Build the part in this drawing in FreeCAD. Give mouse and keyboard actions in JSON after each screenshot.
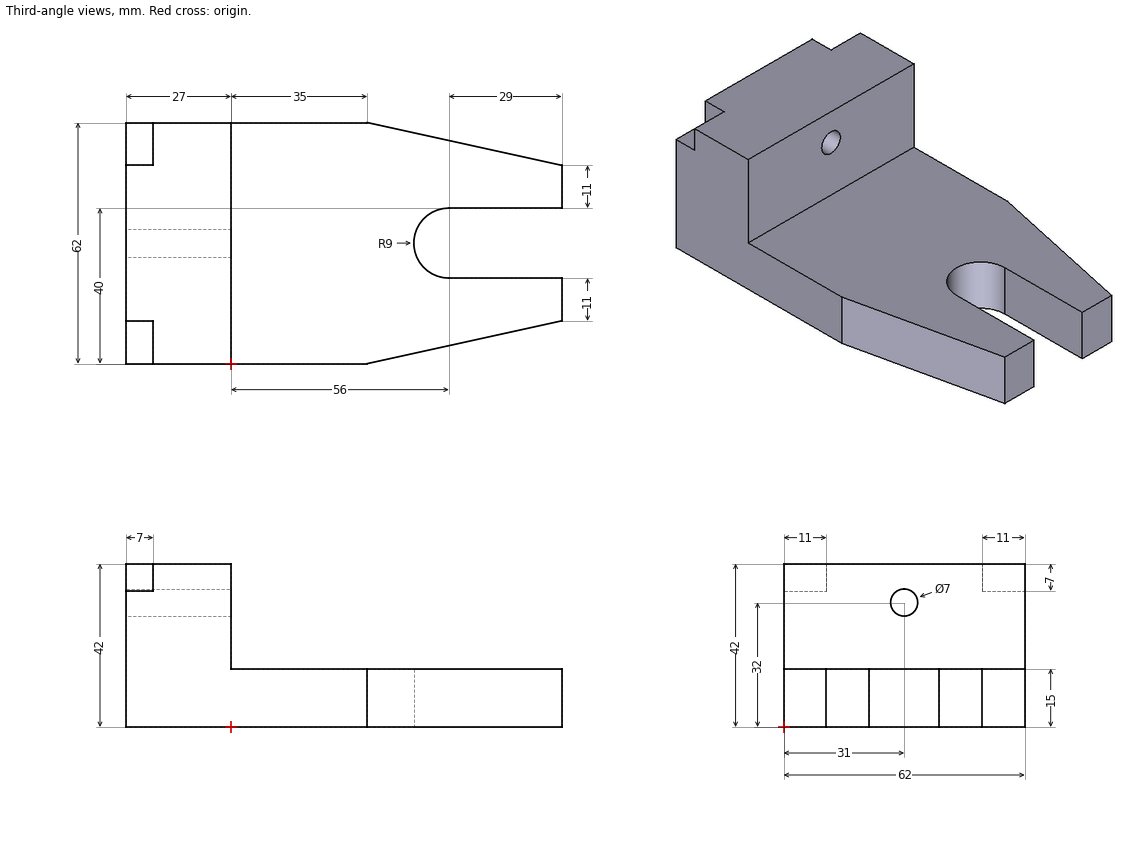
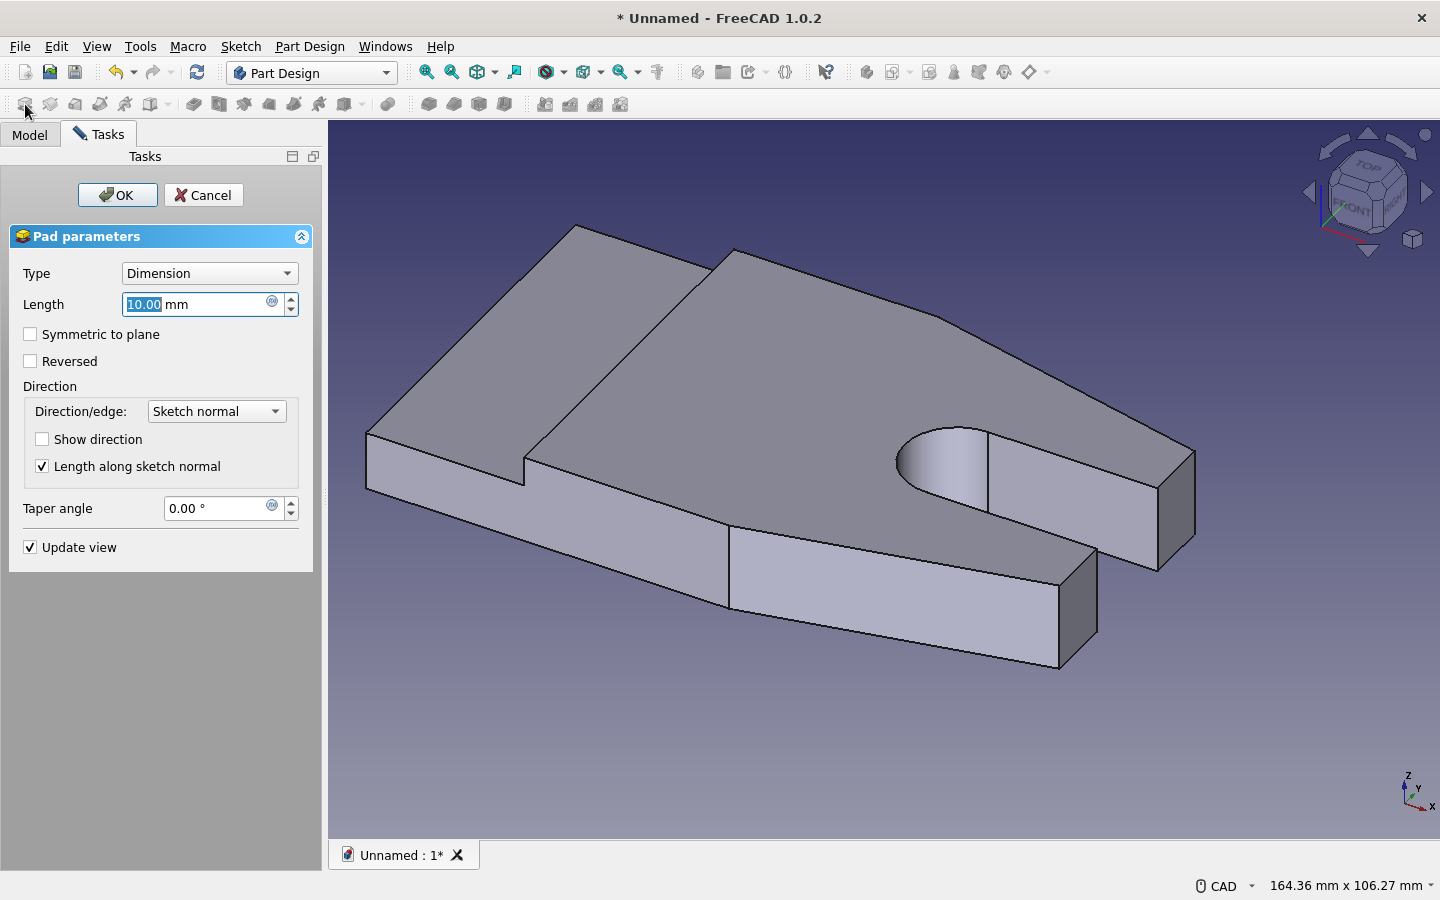
{"action": "type", "text": "42"}
{"action": "key", "text": "Tab"}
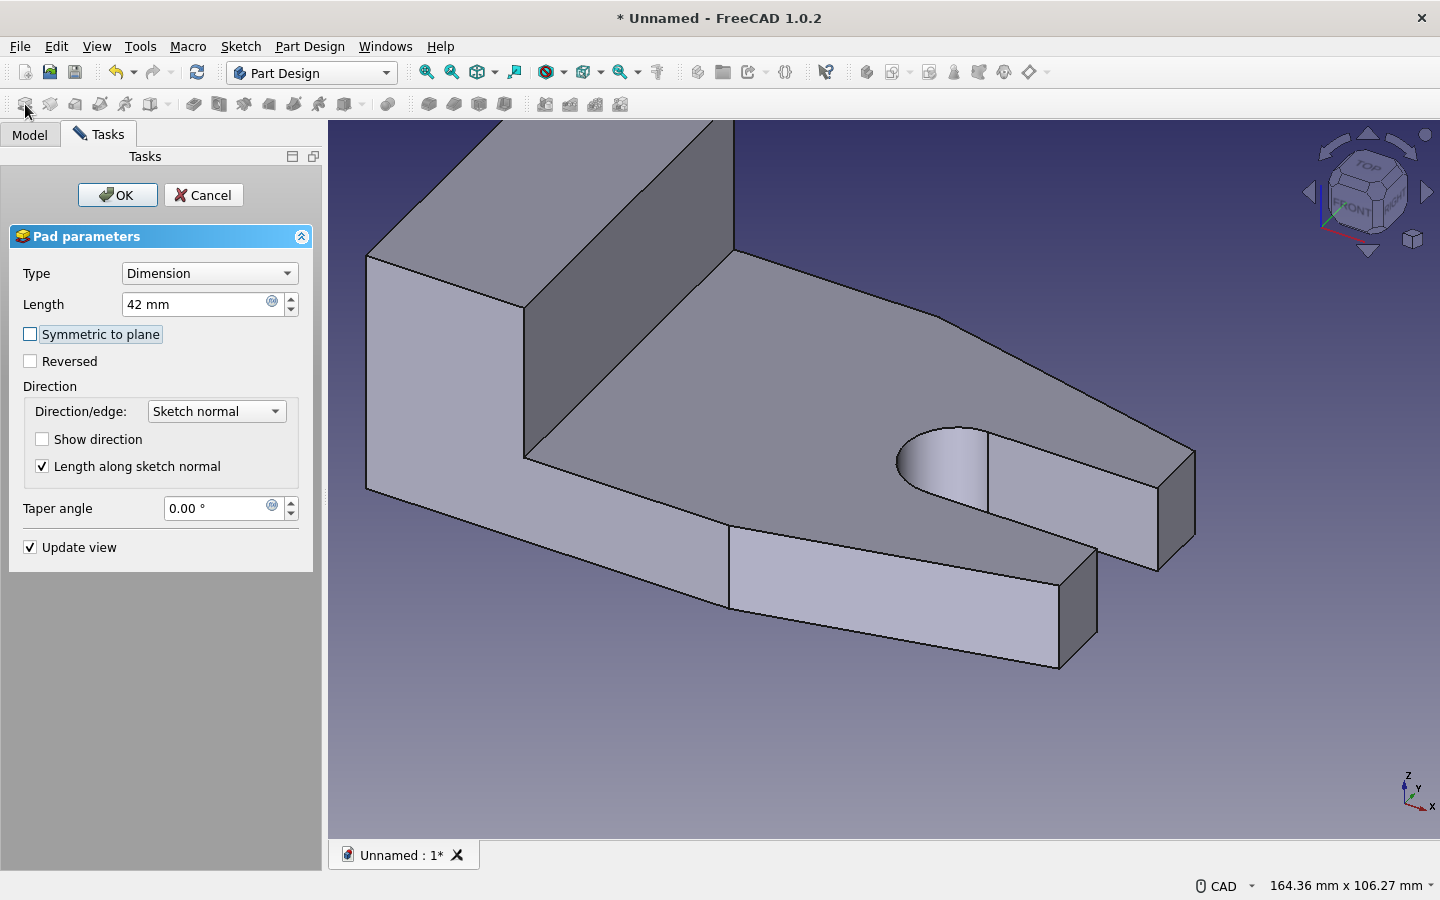
{"action": "left_click", "coordinate": [118, 195]}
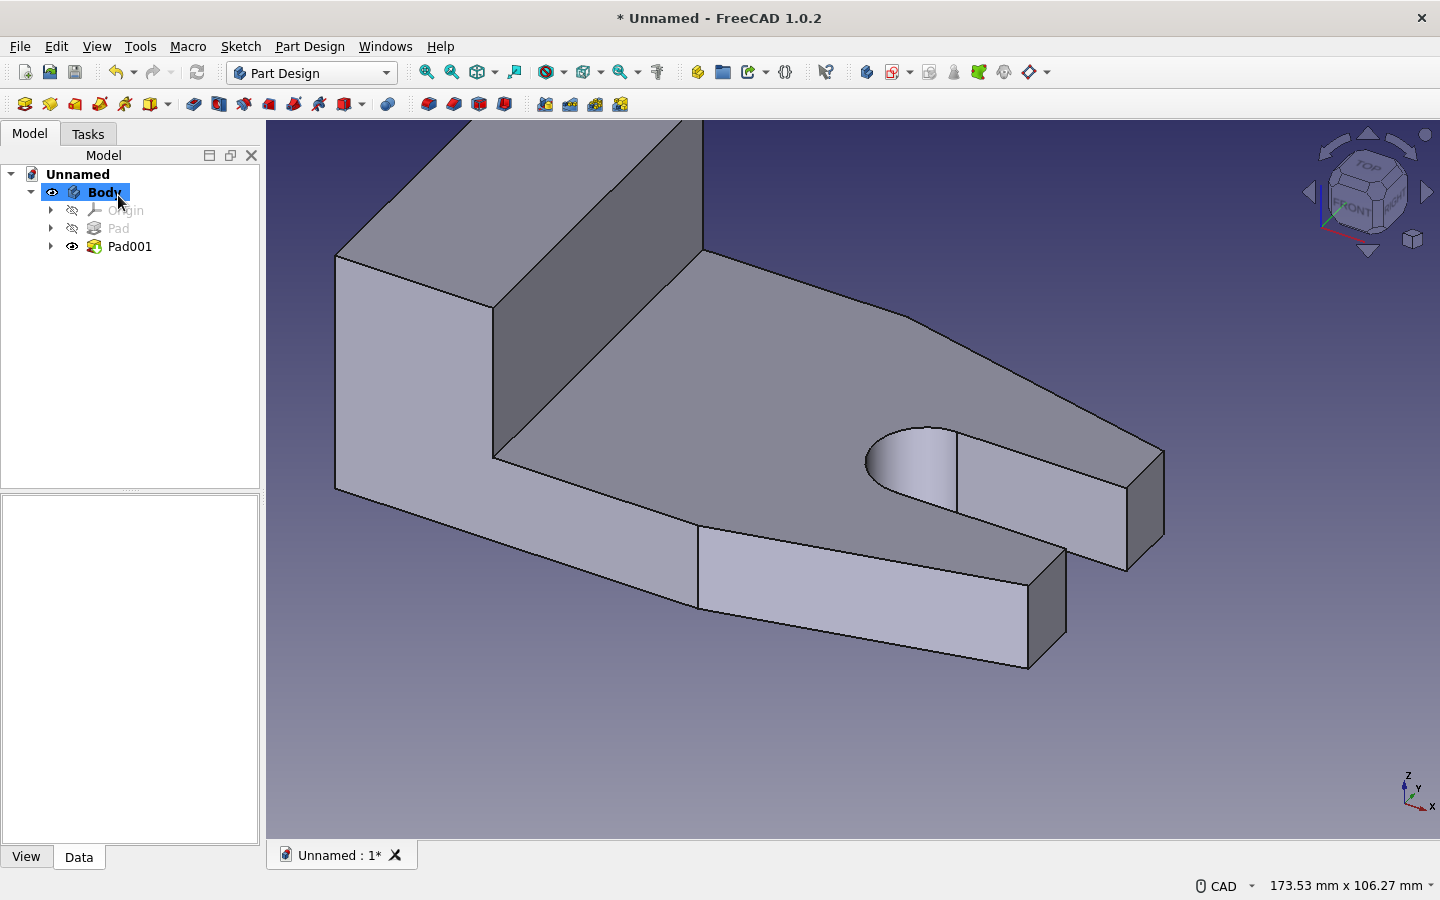
{"action": "left_click", "coordinate": [427, 72]}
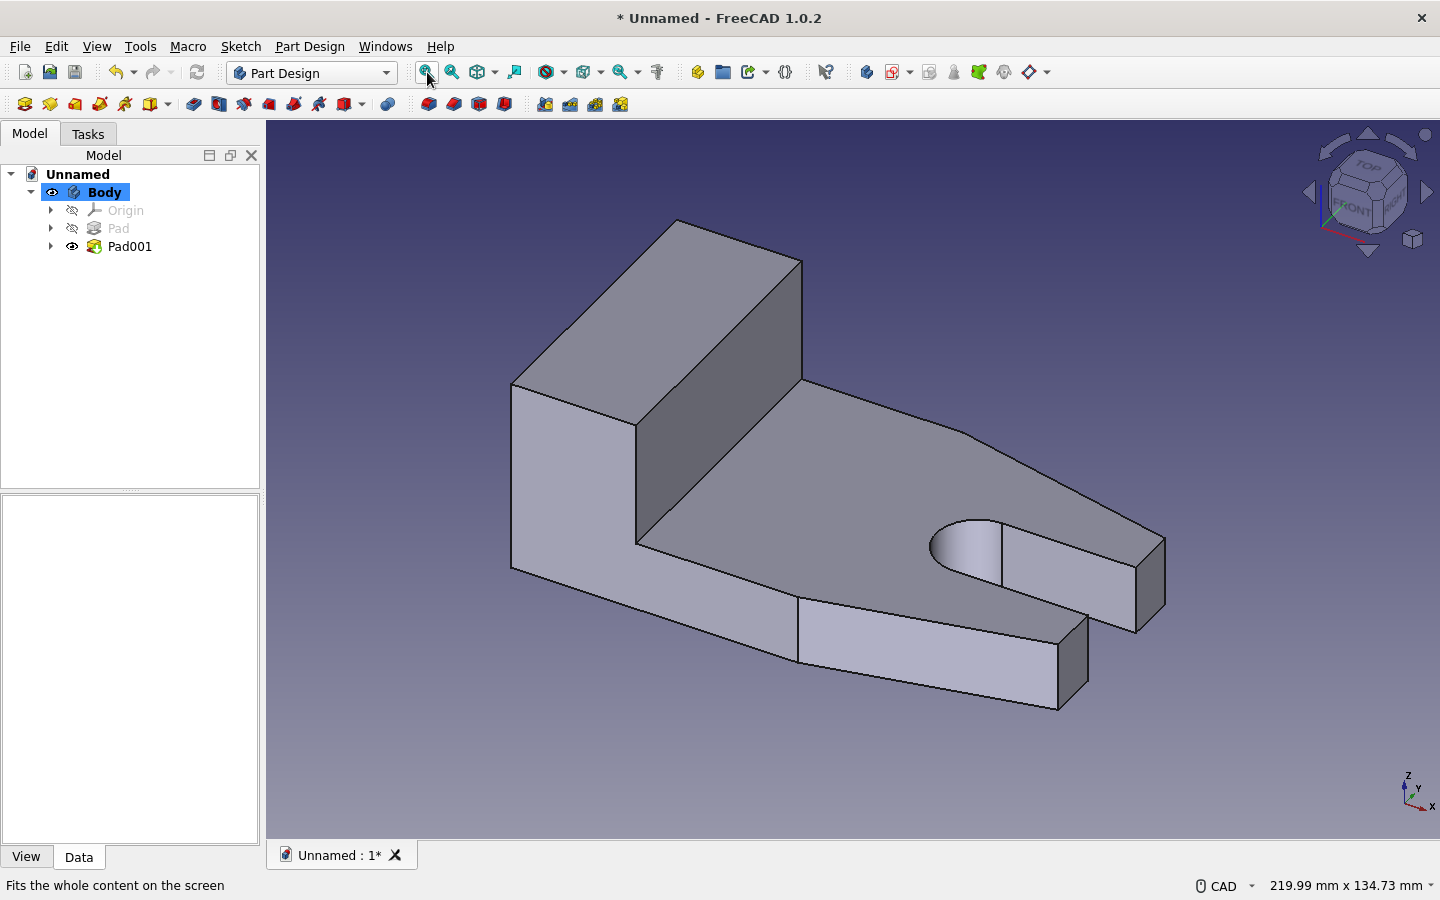
{"action": "key", "text": "6"}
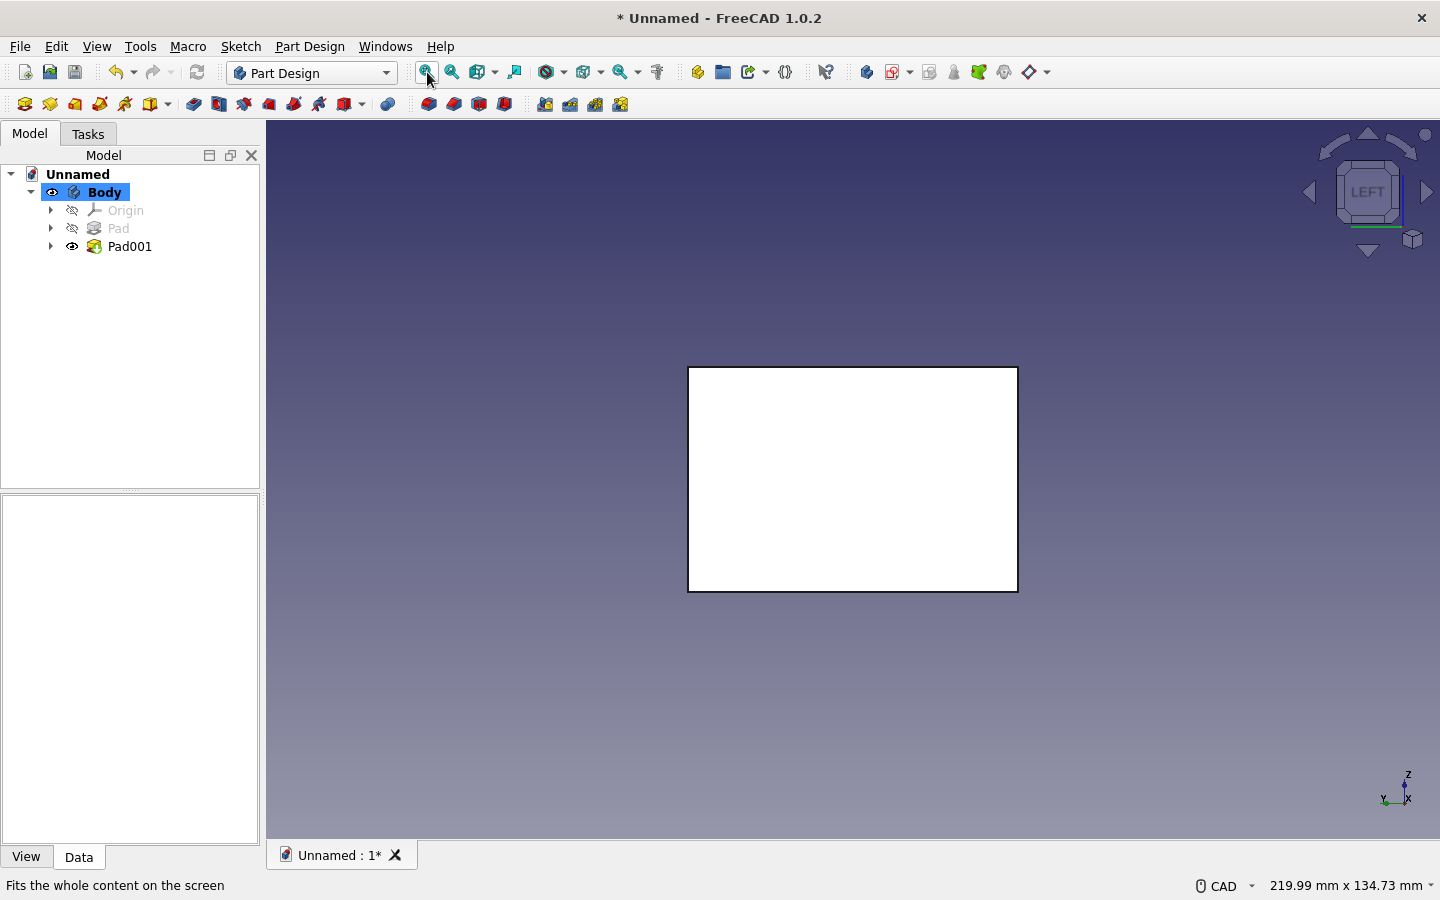
{"action": "left_click", "coordinate": [427, 72]}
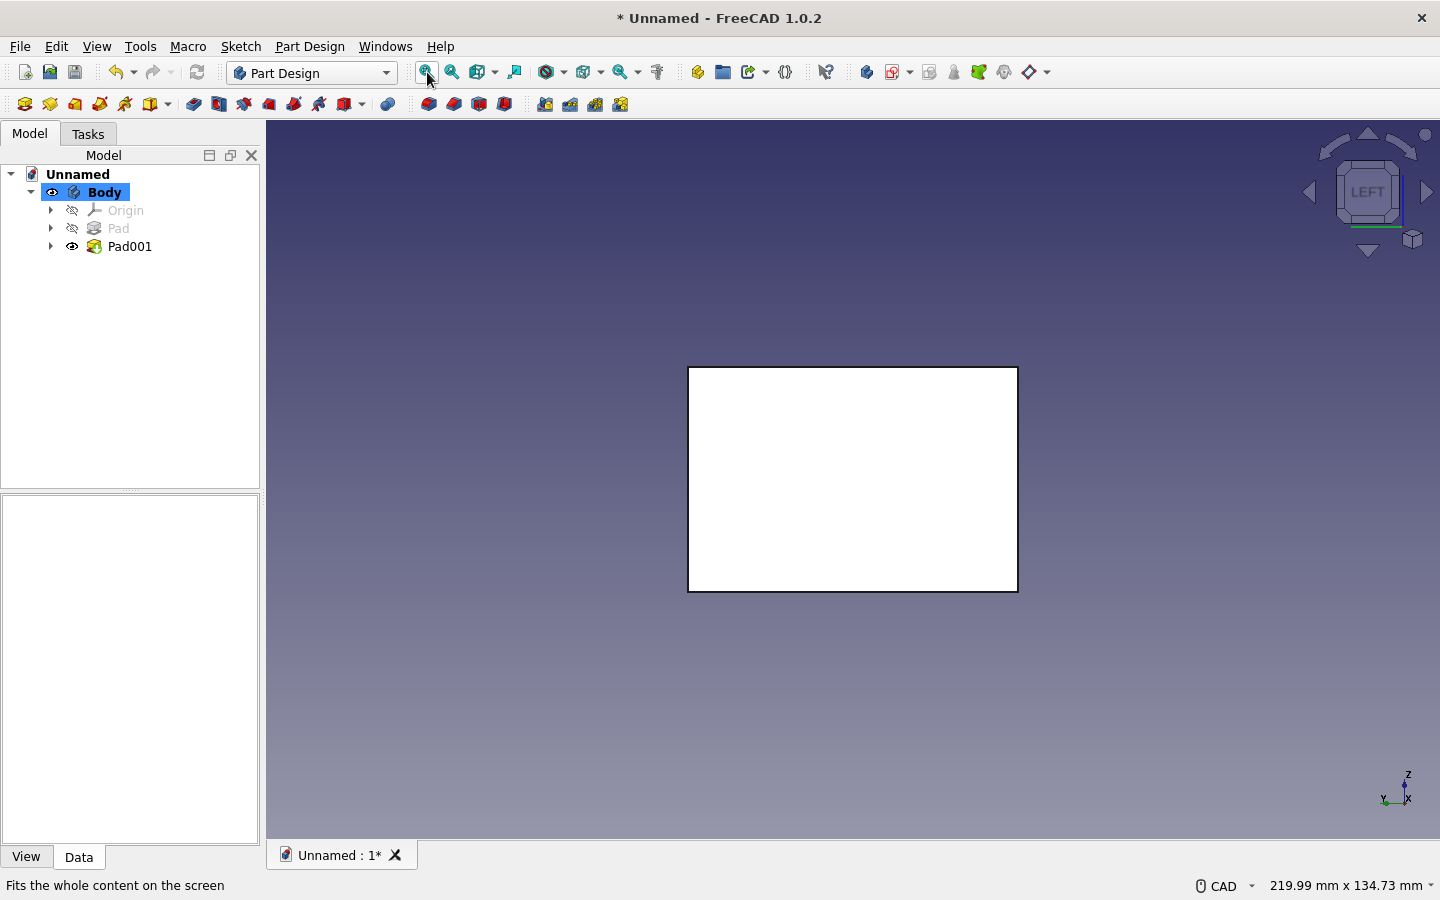
{"action": "left_click", "coordinate": [806, 478]}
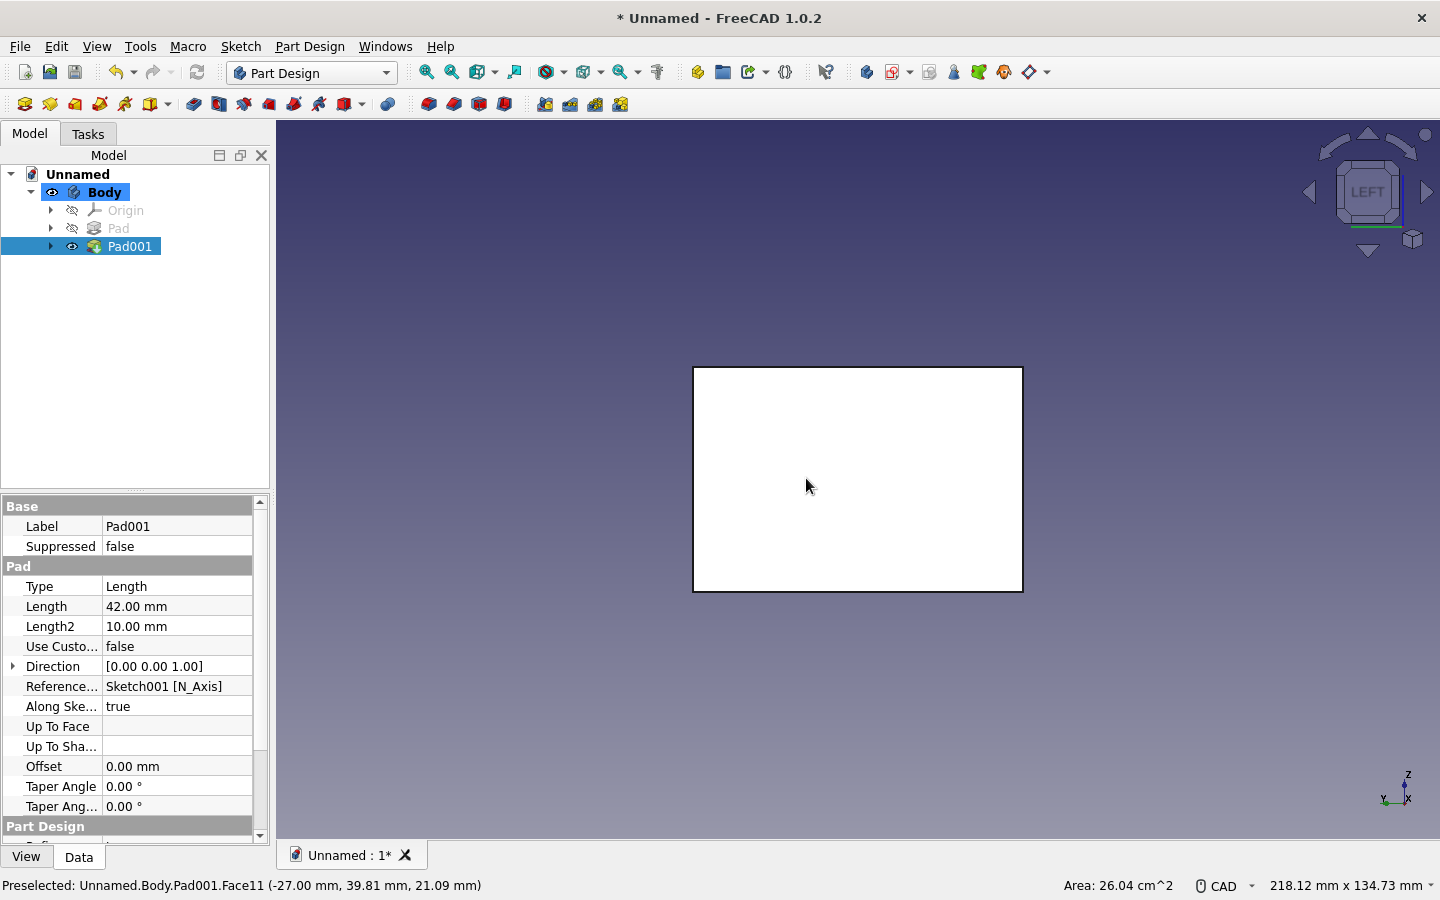
{"action": "left_click", "coordinate": [892, 72]}